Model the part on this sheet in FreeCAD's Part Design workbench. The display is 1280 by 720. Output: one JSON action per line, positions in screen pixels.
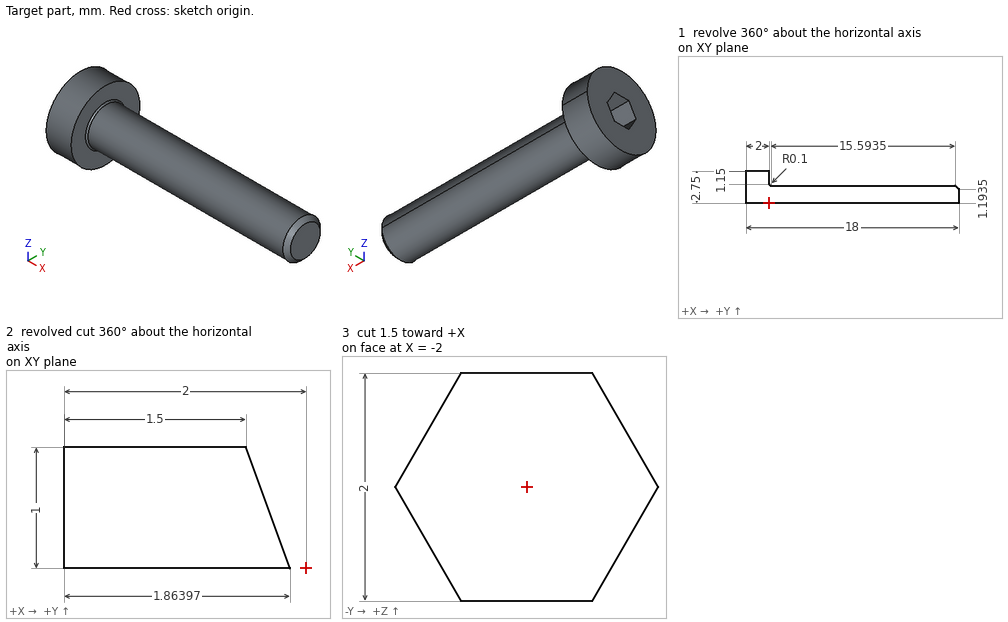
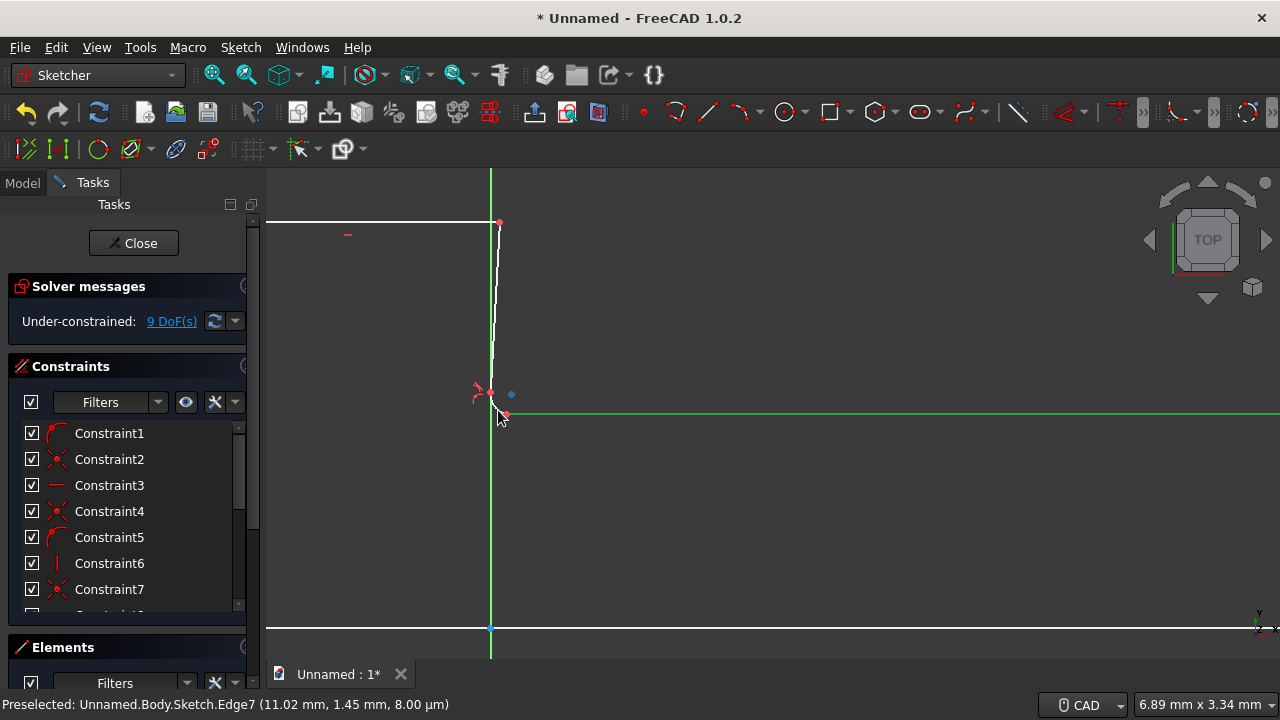
{"action": "left_click", "coordinate": [495, 407]}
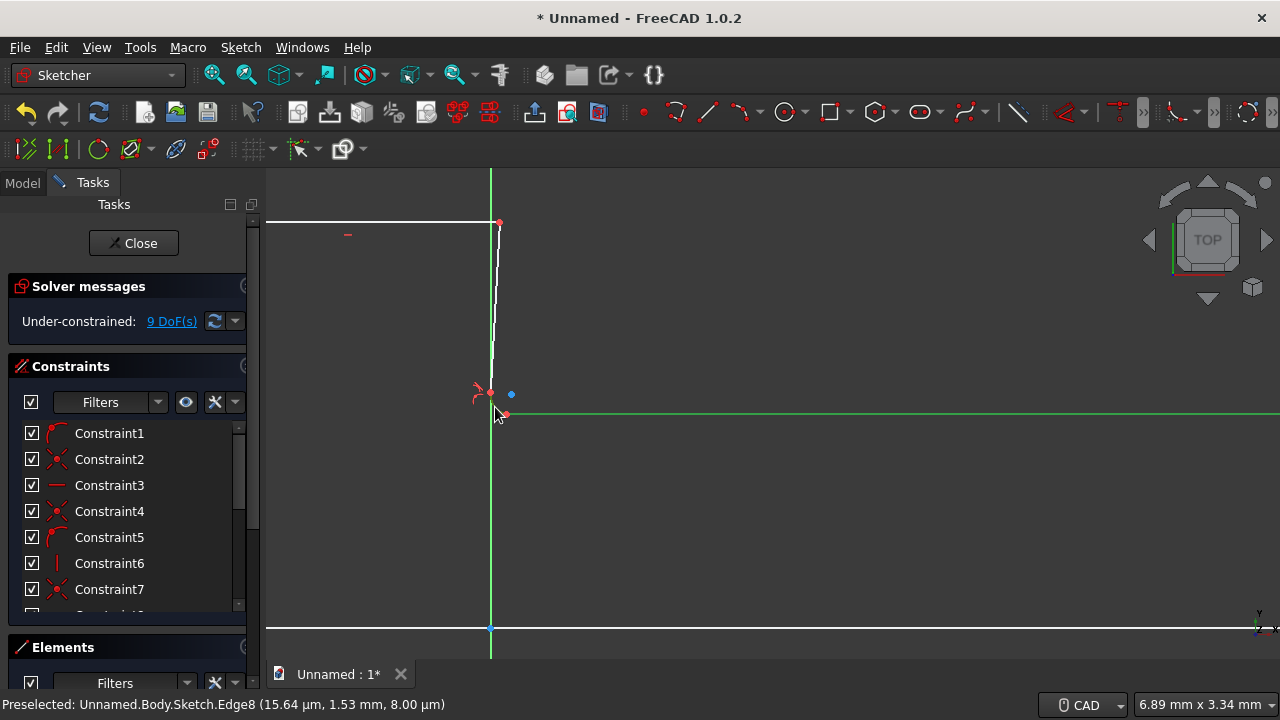
{"action": "key", "text": "t"}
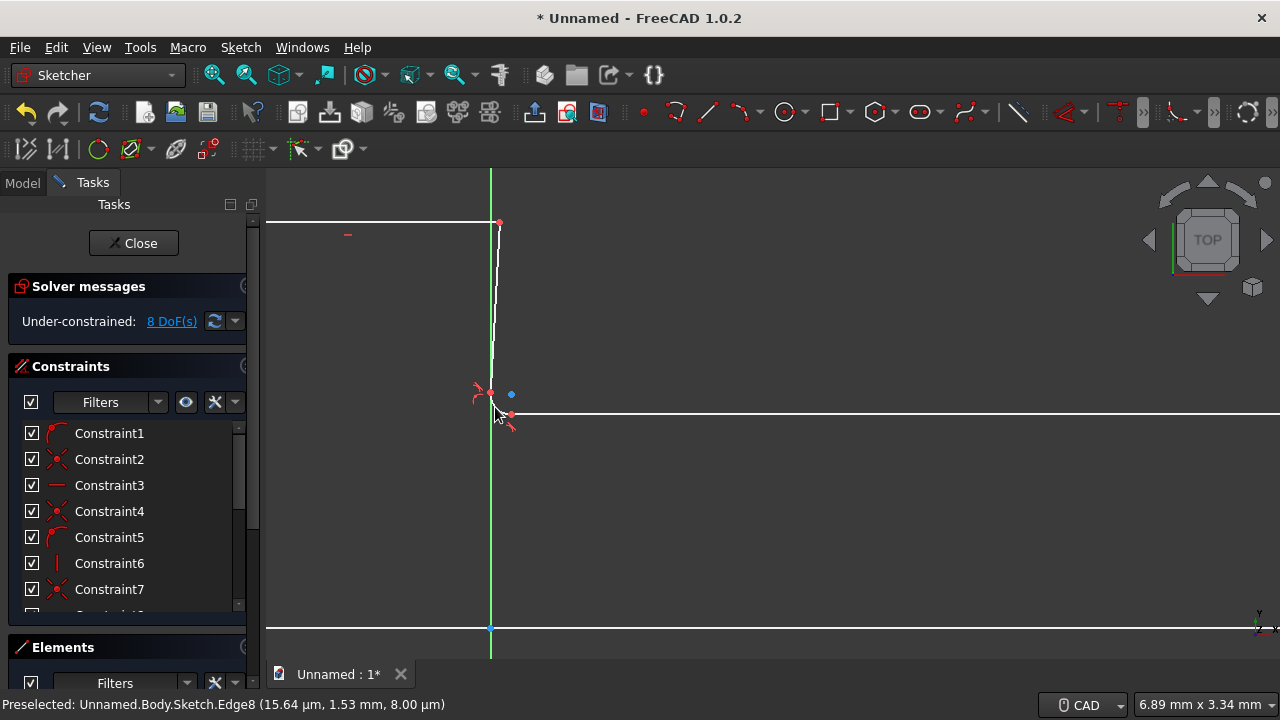
{"action": "scroll", "coordinate": [498, 410], "scroll_direction": "down", "scroll_amount": 8}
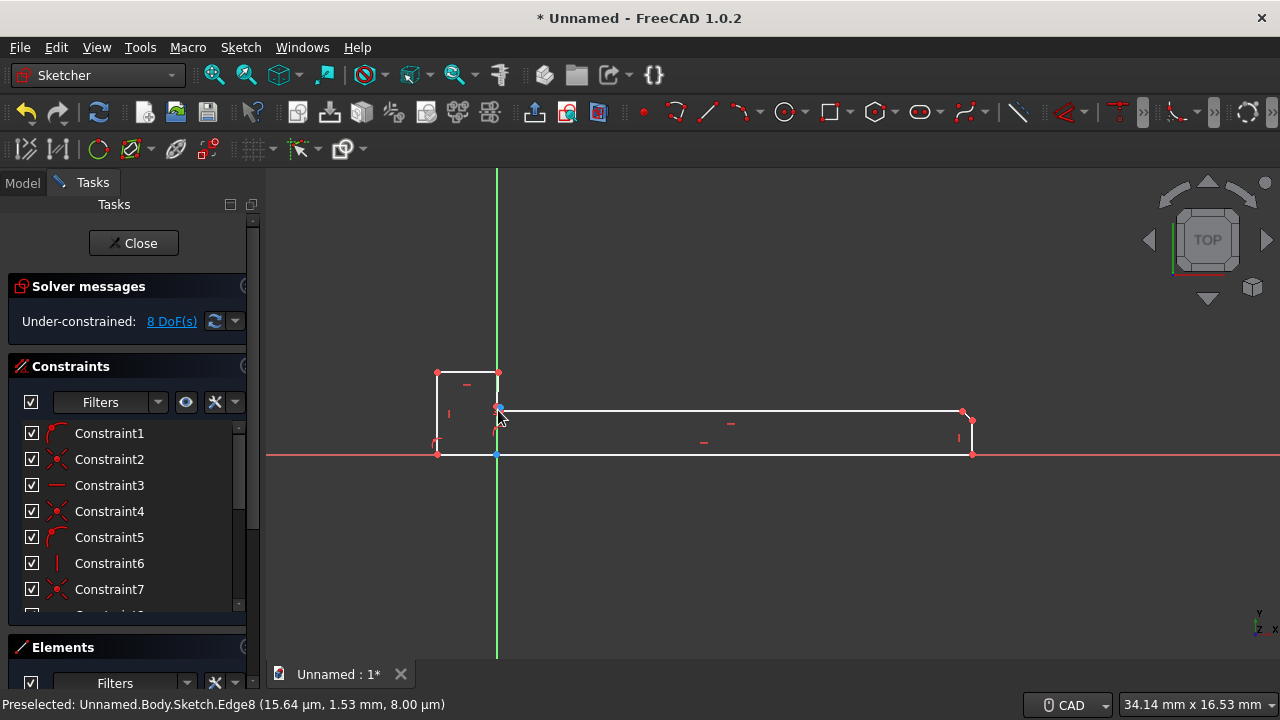
{"action": "scroll", "coordinate": [497, 397], "scroll_direction": "up", "scroll_amount": 2}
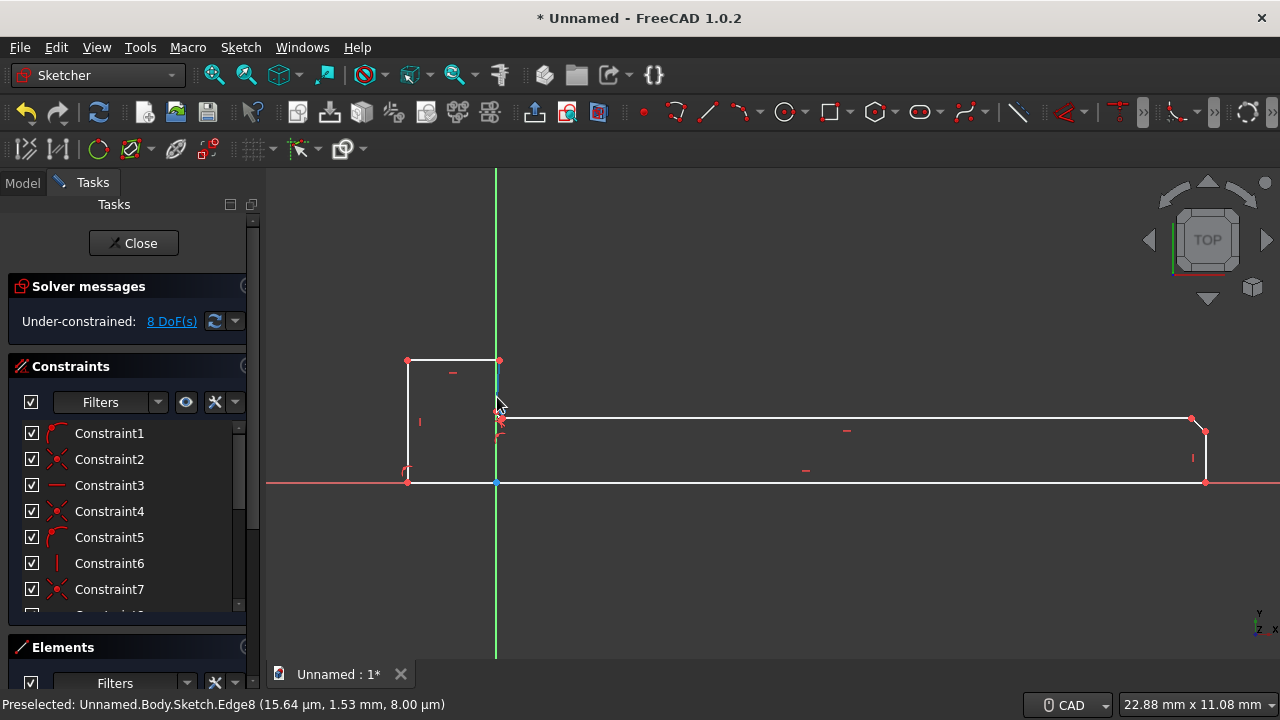
{"action": "left_click", "coordinate": [497, 396]}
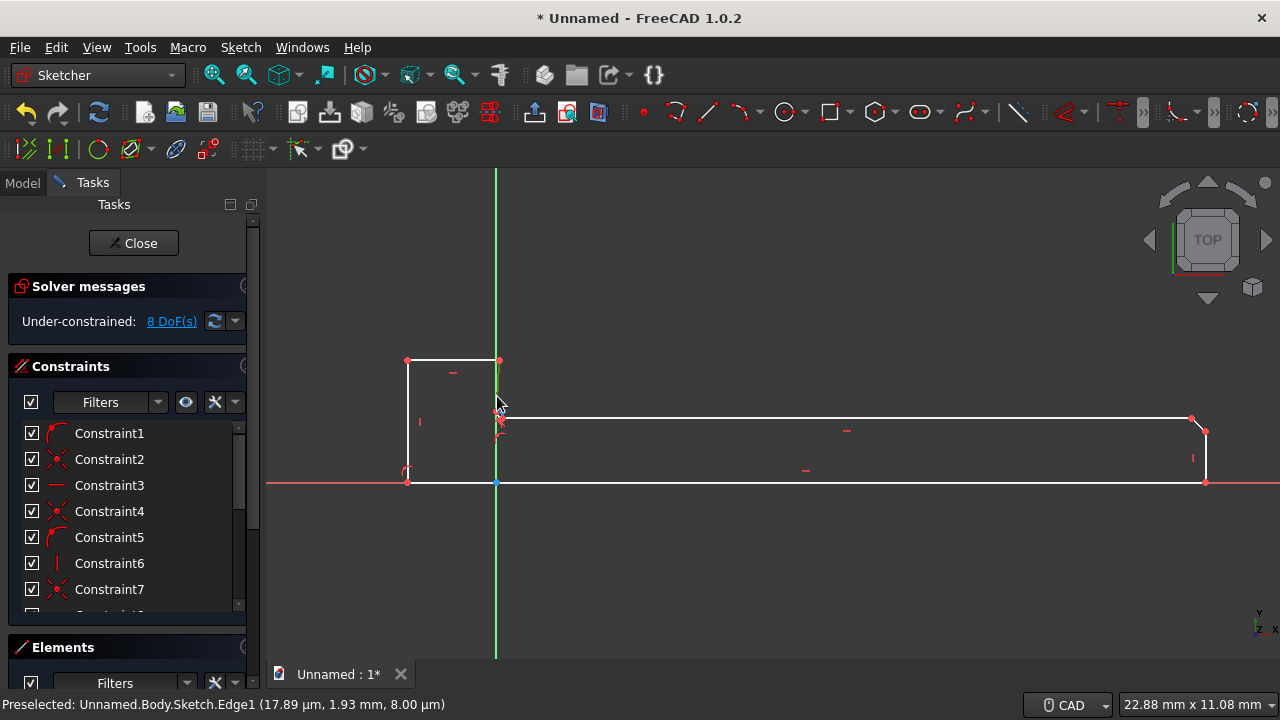
{"action": "key", "text": "v"}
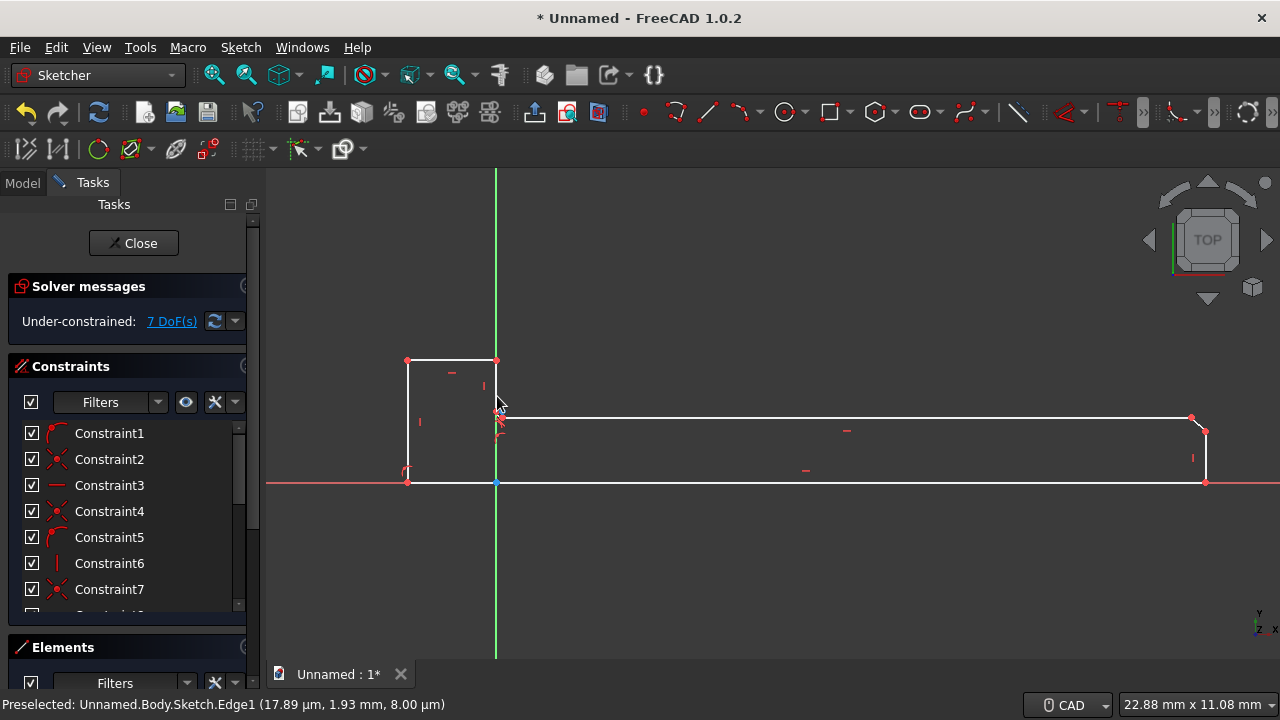
{"action": "left_click", "coordinate": [1064, 112]}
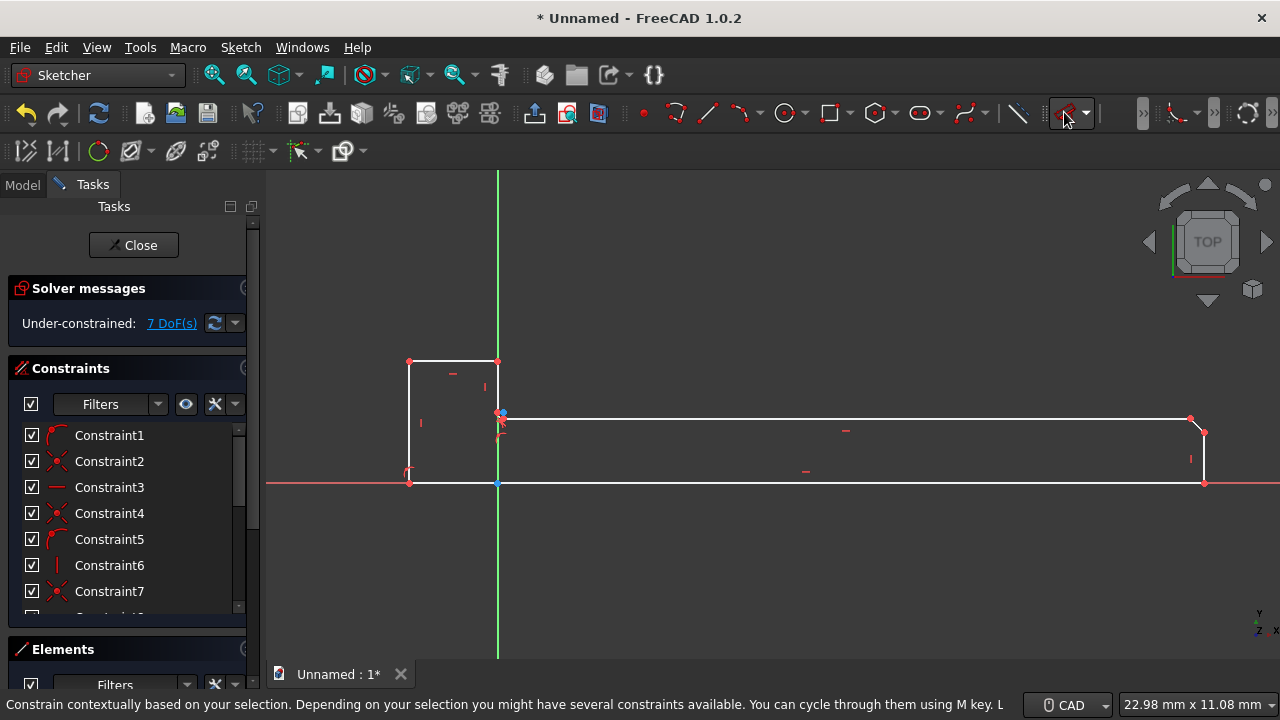
{"action": "scroll", "coordinate": [499, 417], "scroll_direction": "up", "scroll_amount": 11}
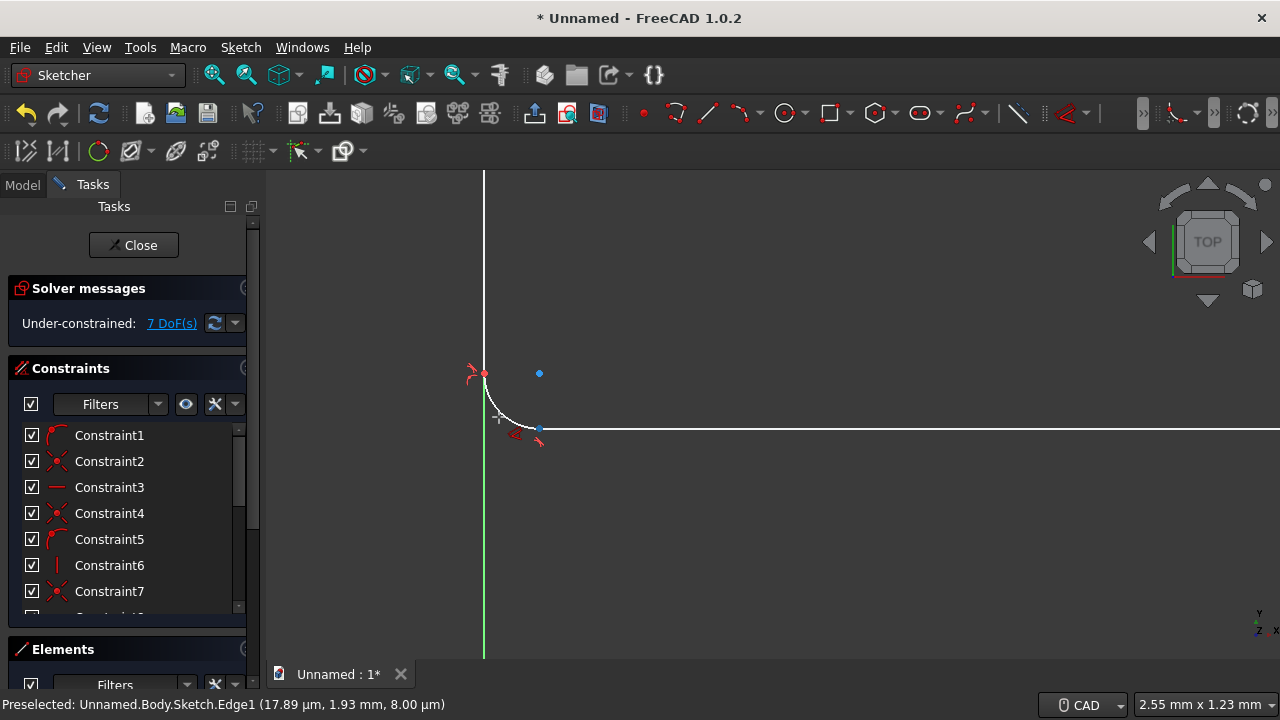
{"action": "left_click", "coordinate": [501, 413]}
{"action": "left_click", "coordinate": [456, 399]}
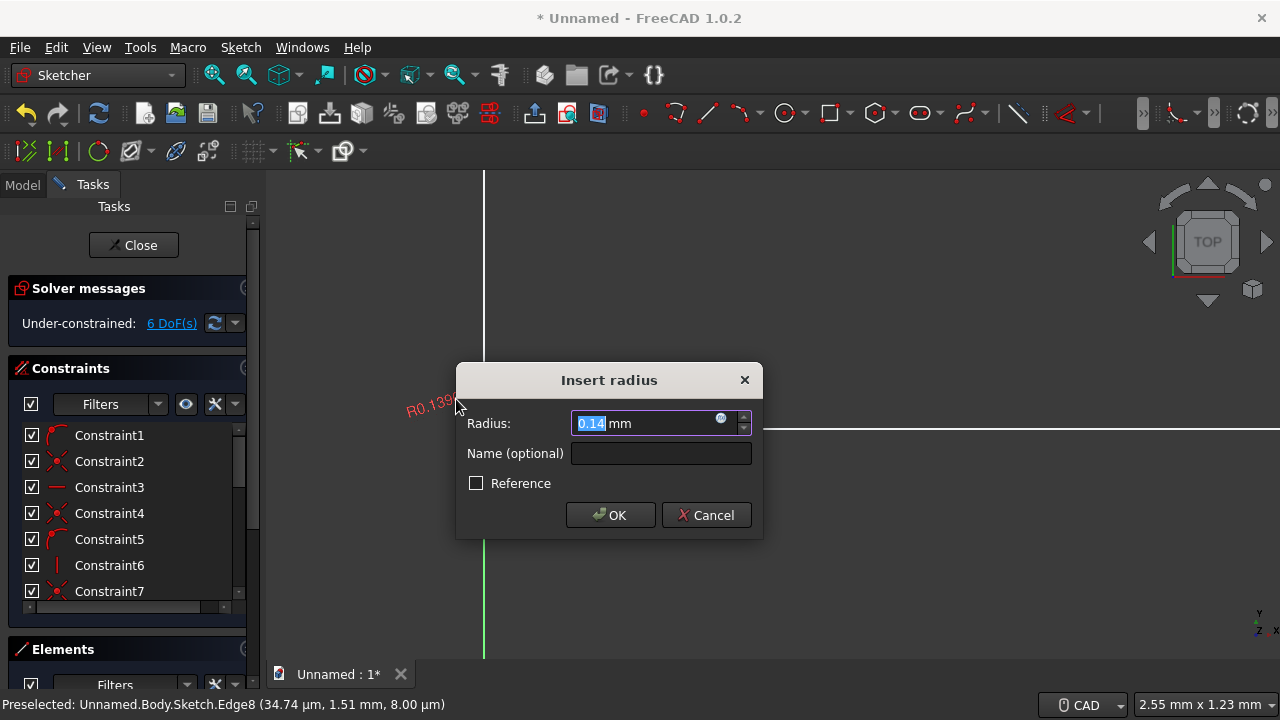
{"action": "type", "text": "0.1"}
{"action": "key", "text": "Return"}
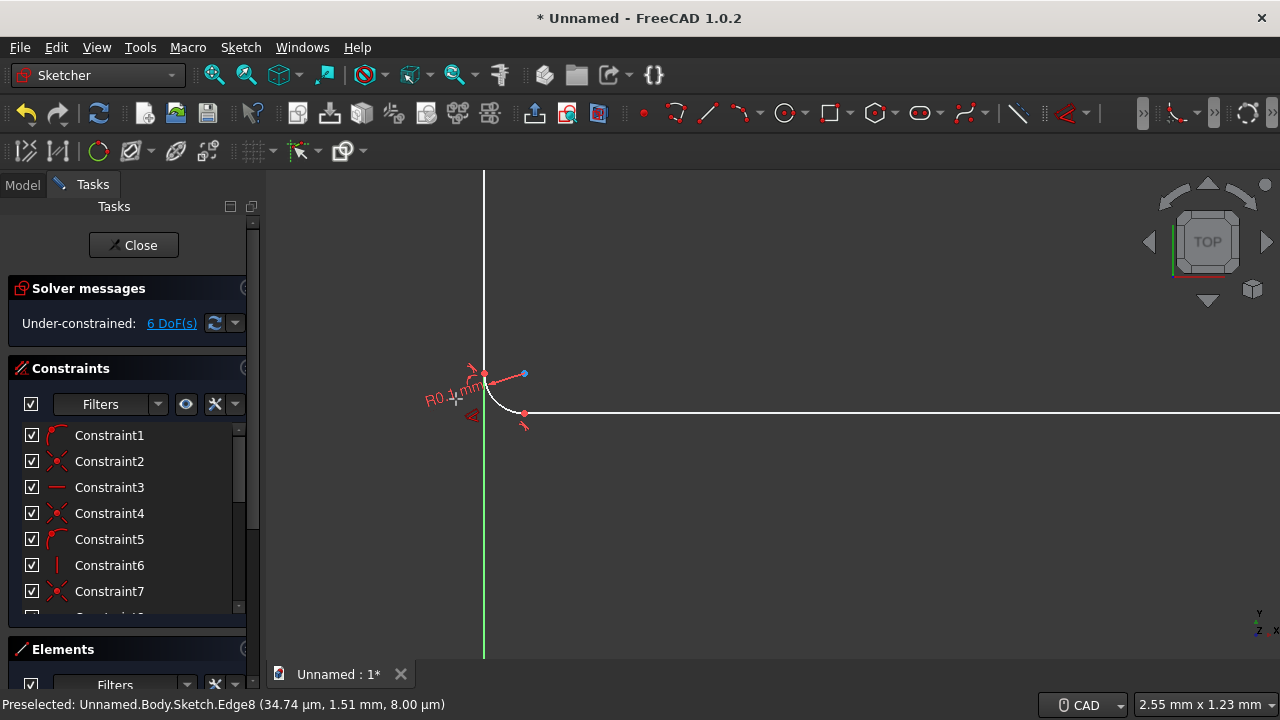
{"action": "scroll", "coordinate": [498, 411], "scroll_direction": "down", "scroll_amount": 13}